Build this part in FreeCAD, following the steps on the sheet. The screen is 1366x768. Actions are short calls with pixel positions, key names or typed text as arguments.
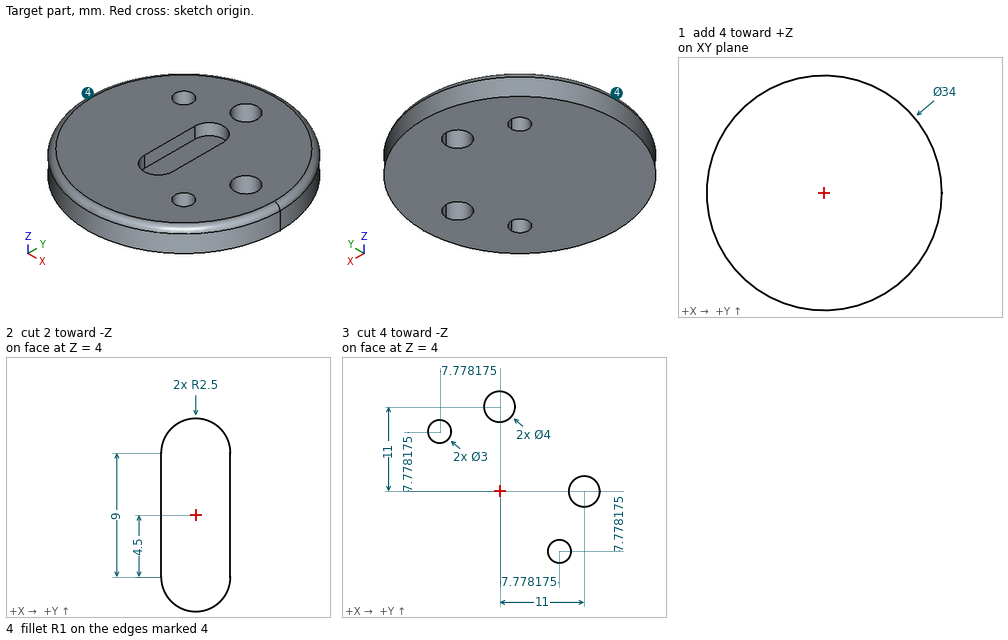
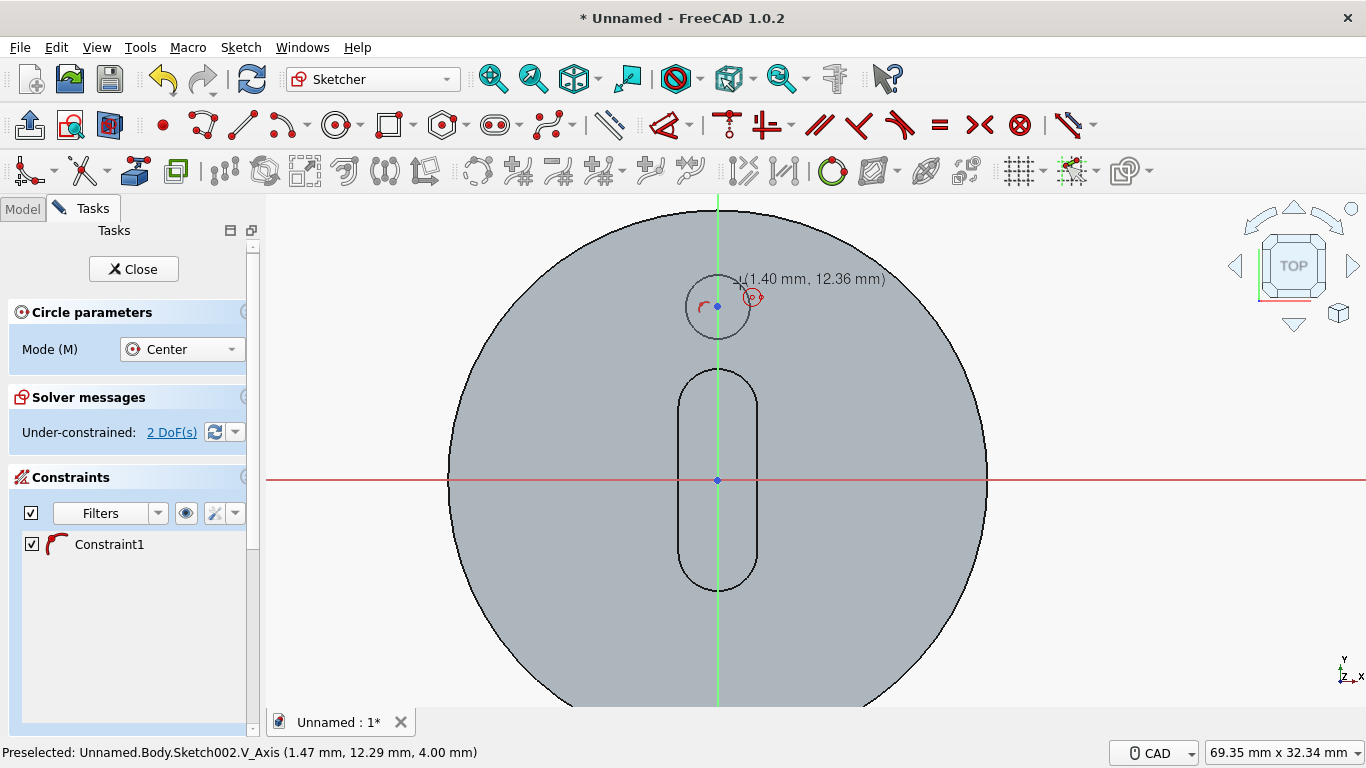
click(892, 480)
click(915, 458)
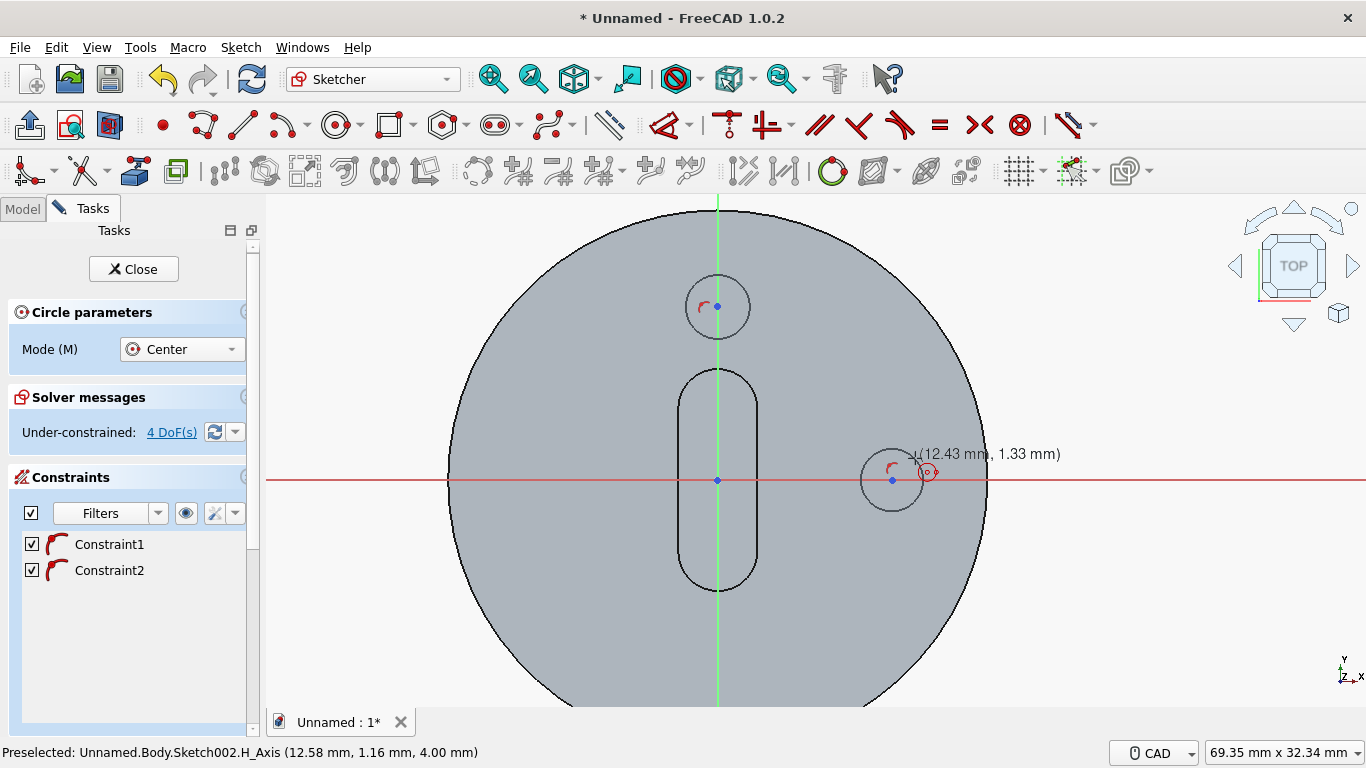
click(594, 357)
click(611, 340)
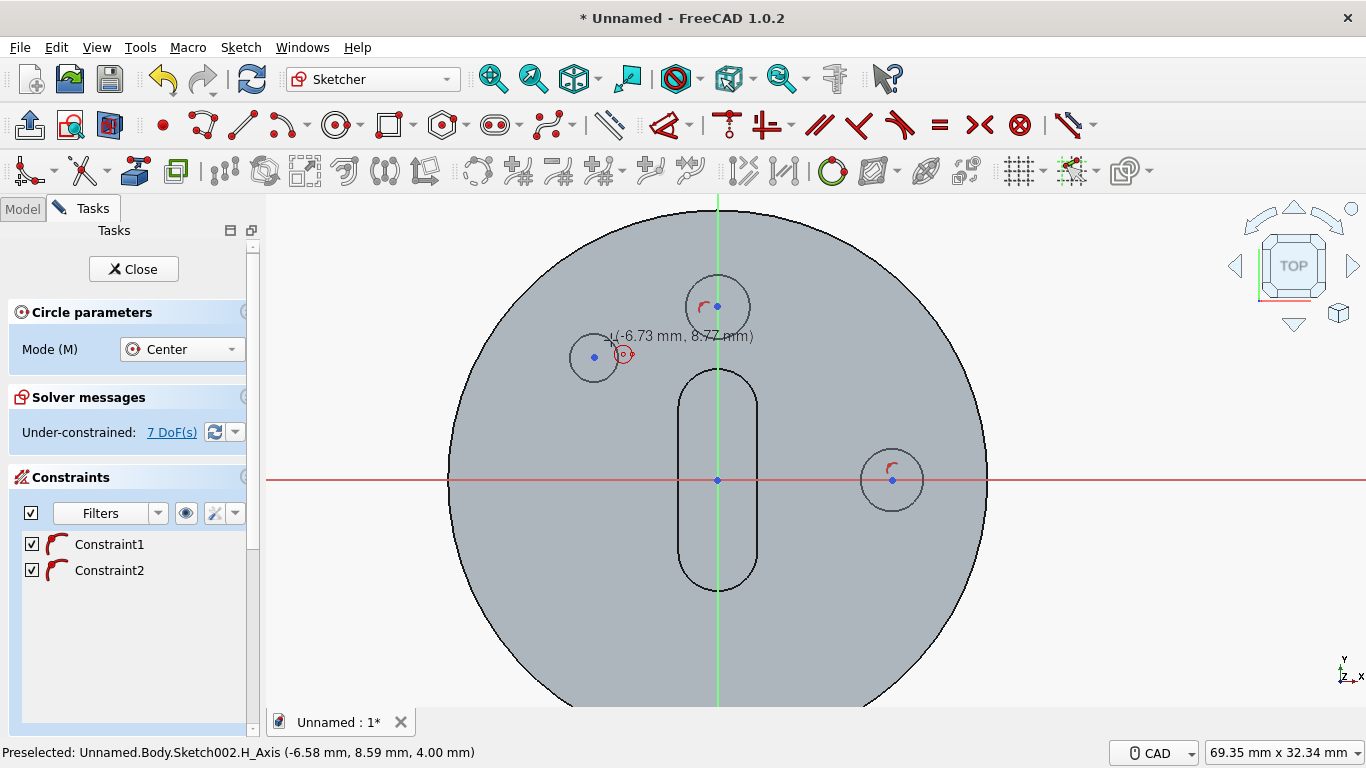
click(841, 603)
click(858, 587)
key(Escape)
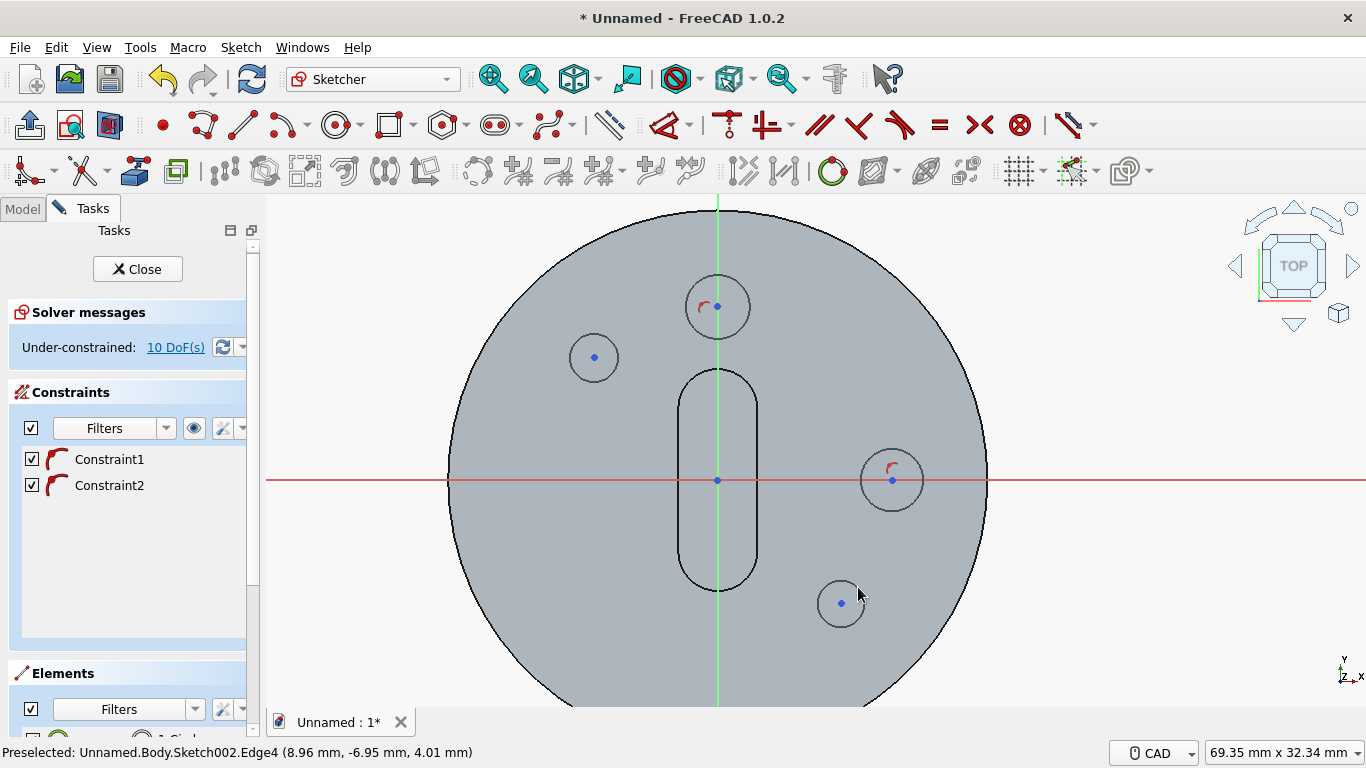
click(740, 284)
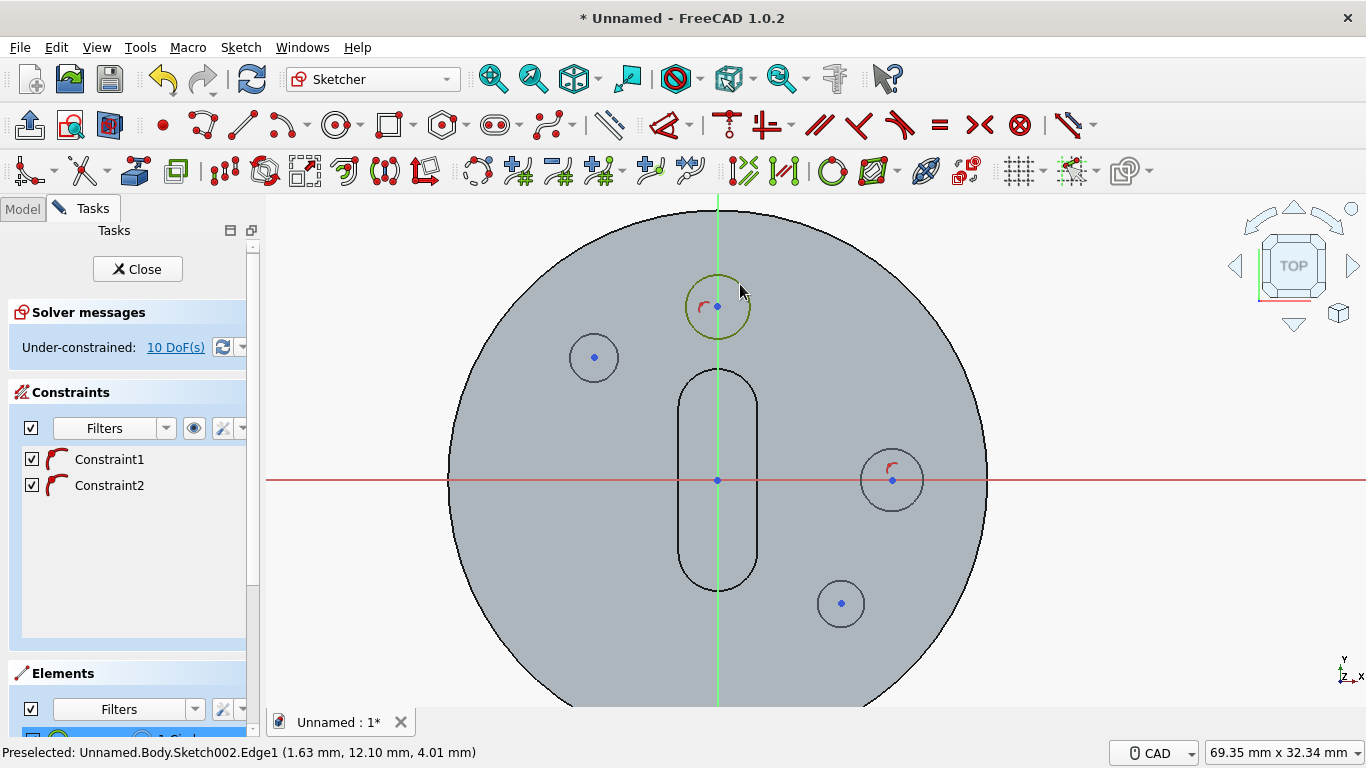
click(914, 458)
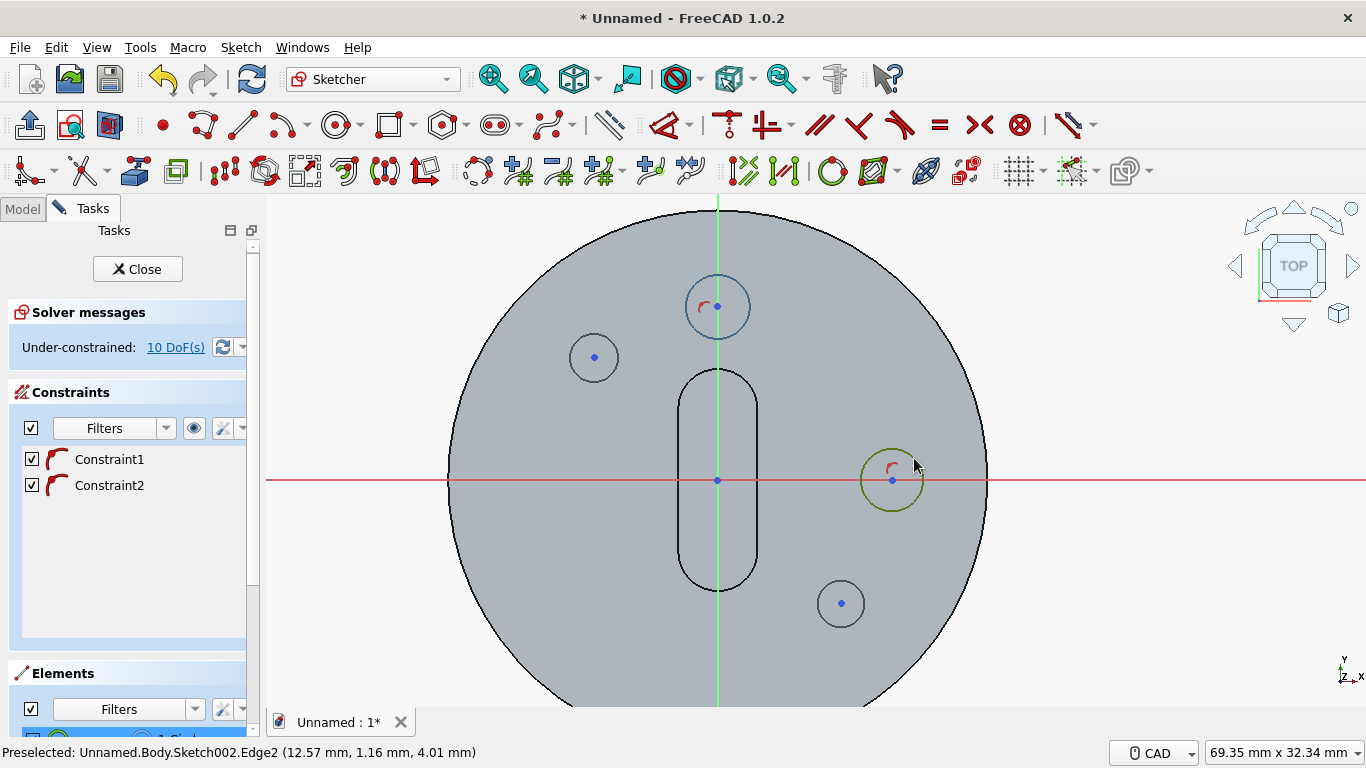
key(e)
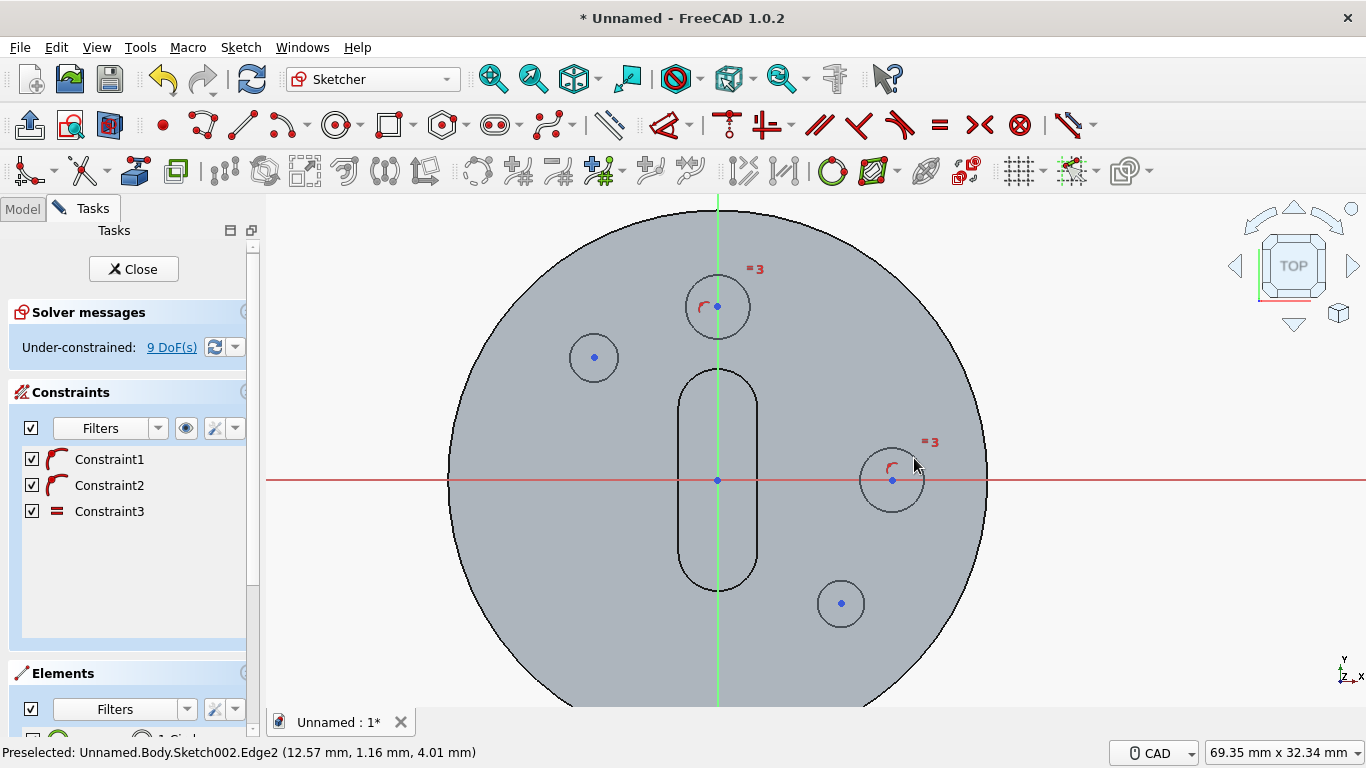
click(611, 341)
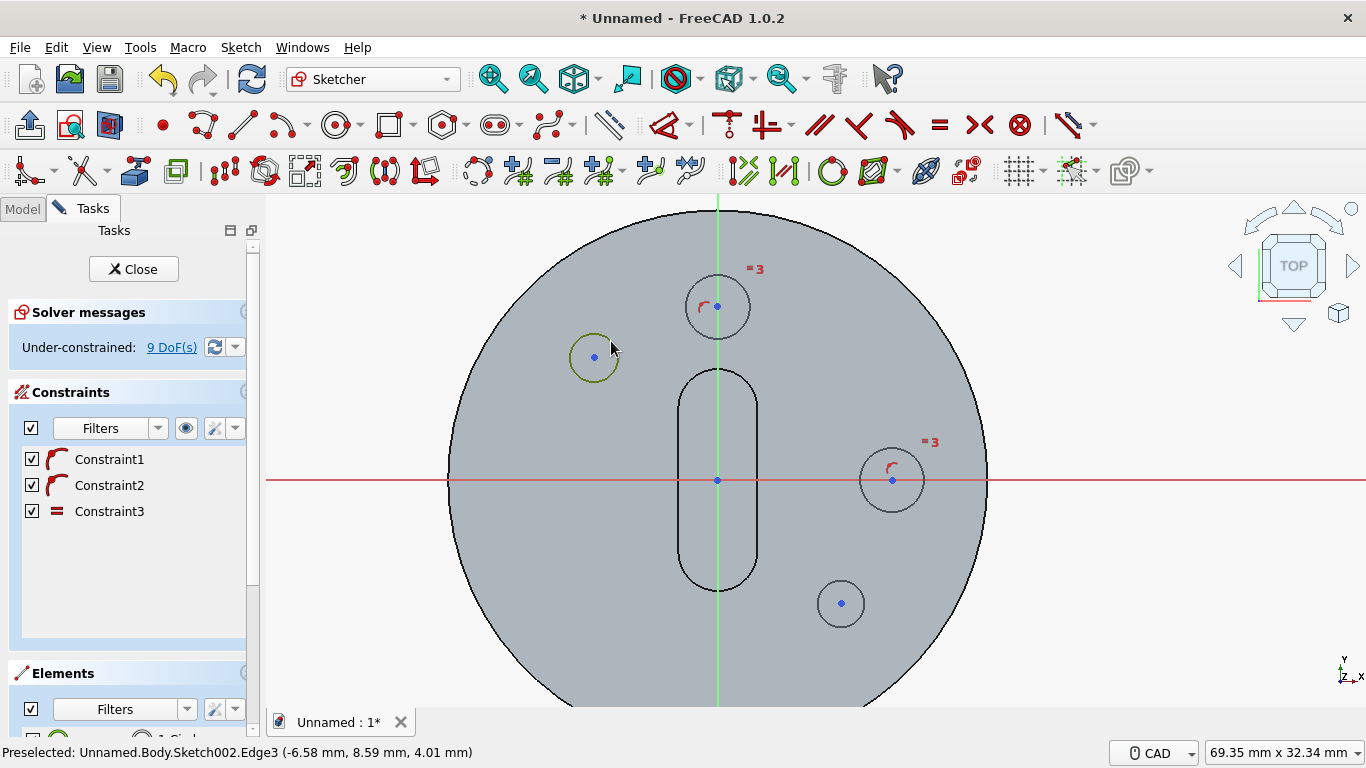
click(857, 587)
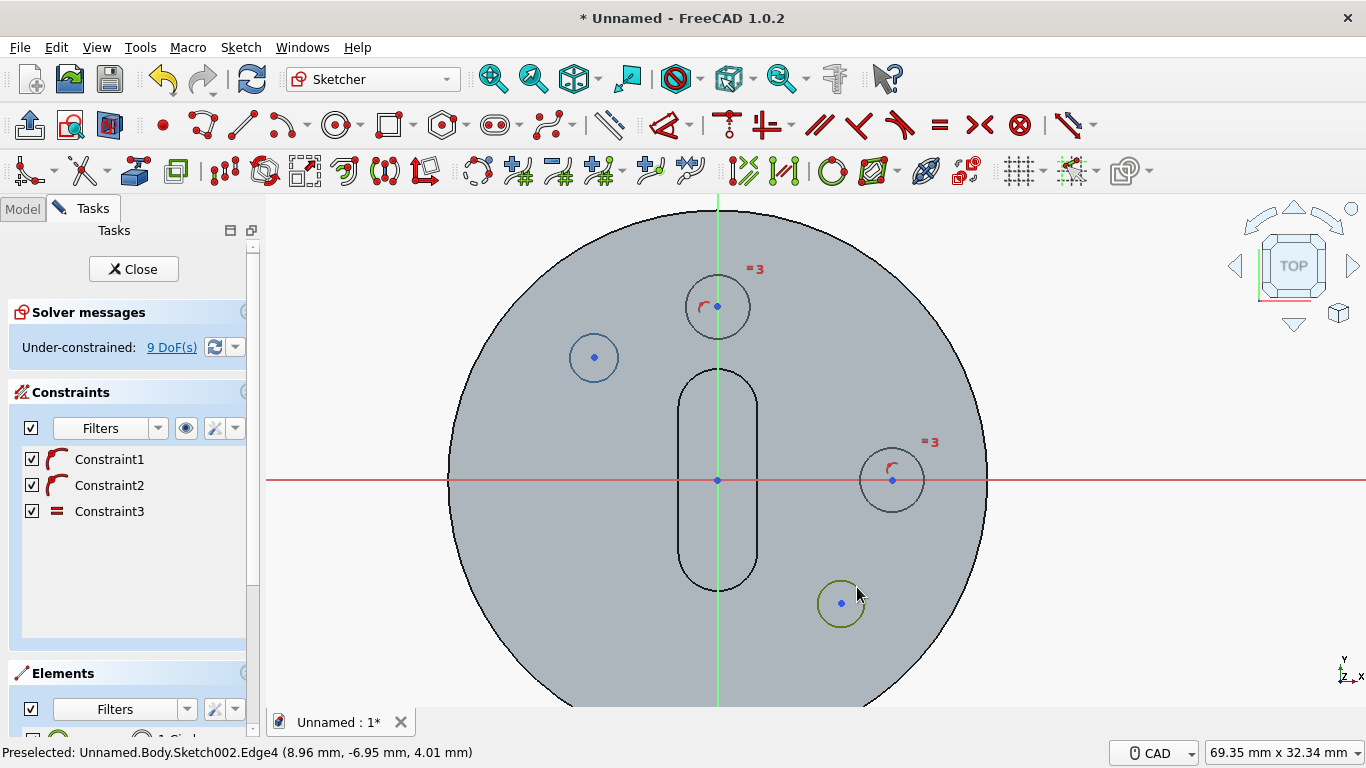
key(e)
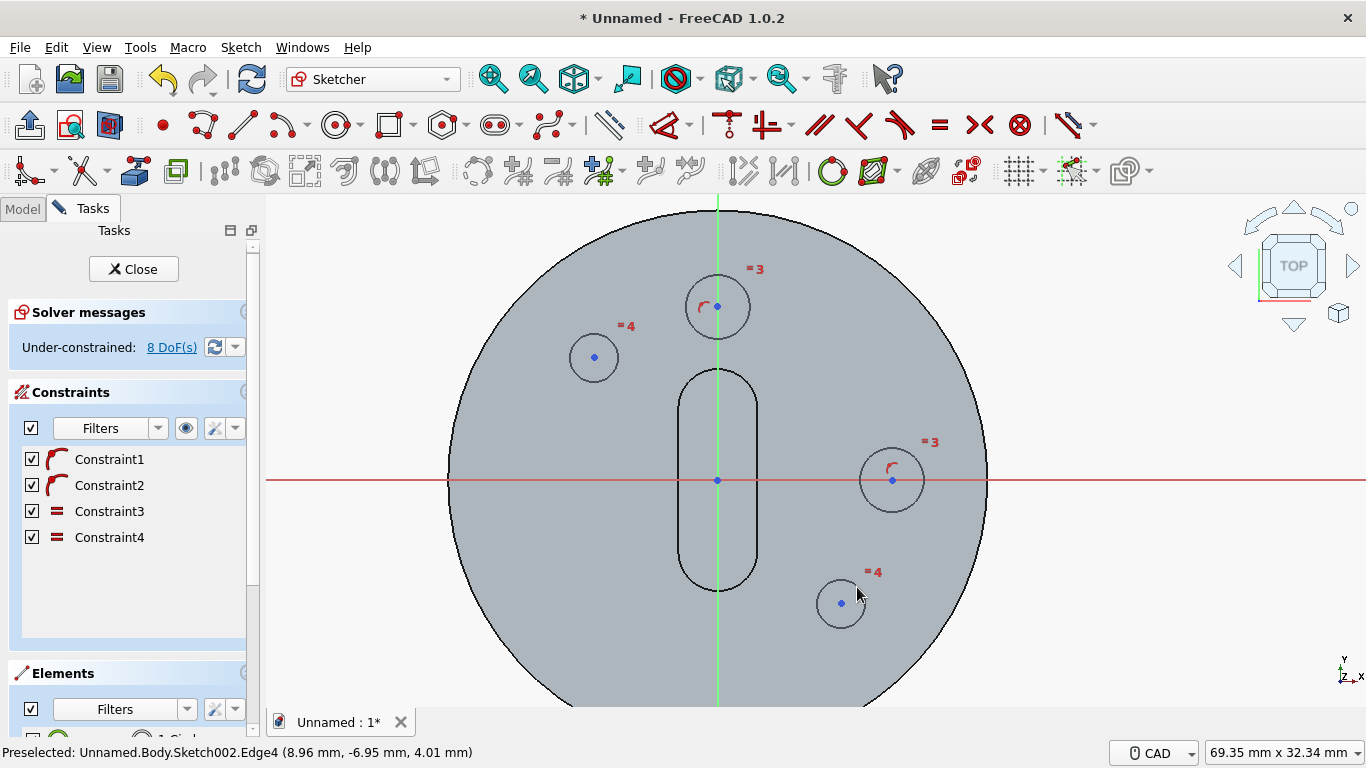
key(d)